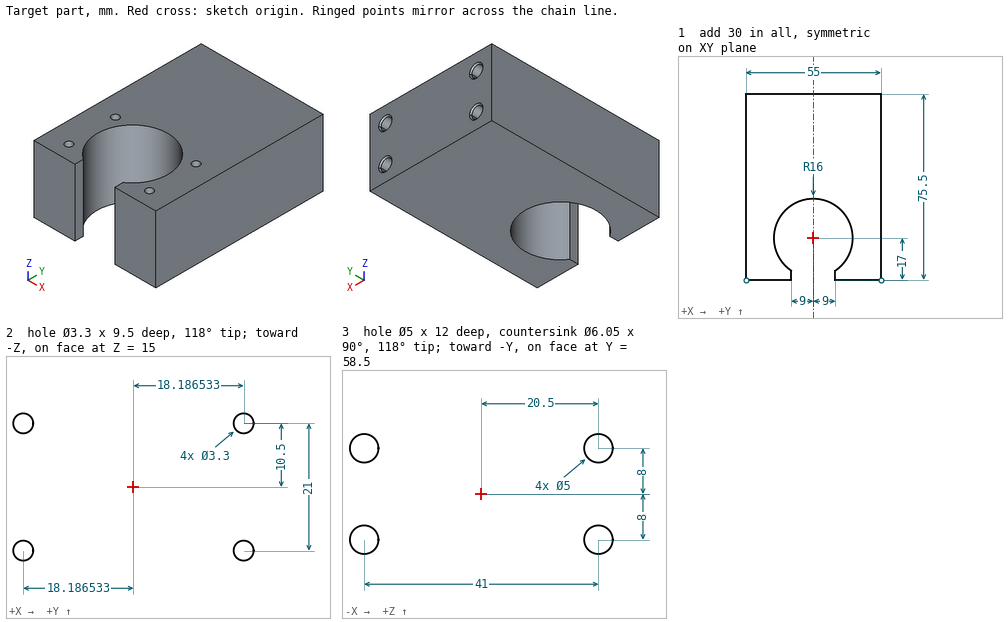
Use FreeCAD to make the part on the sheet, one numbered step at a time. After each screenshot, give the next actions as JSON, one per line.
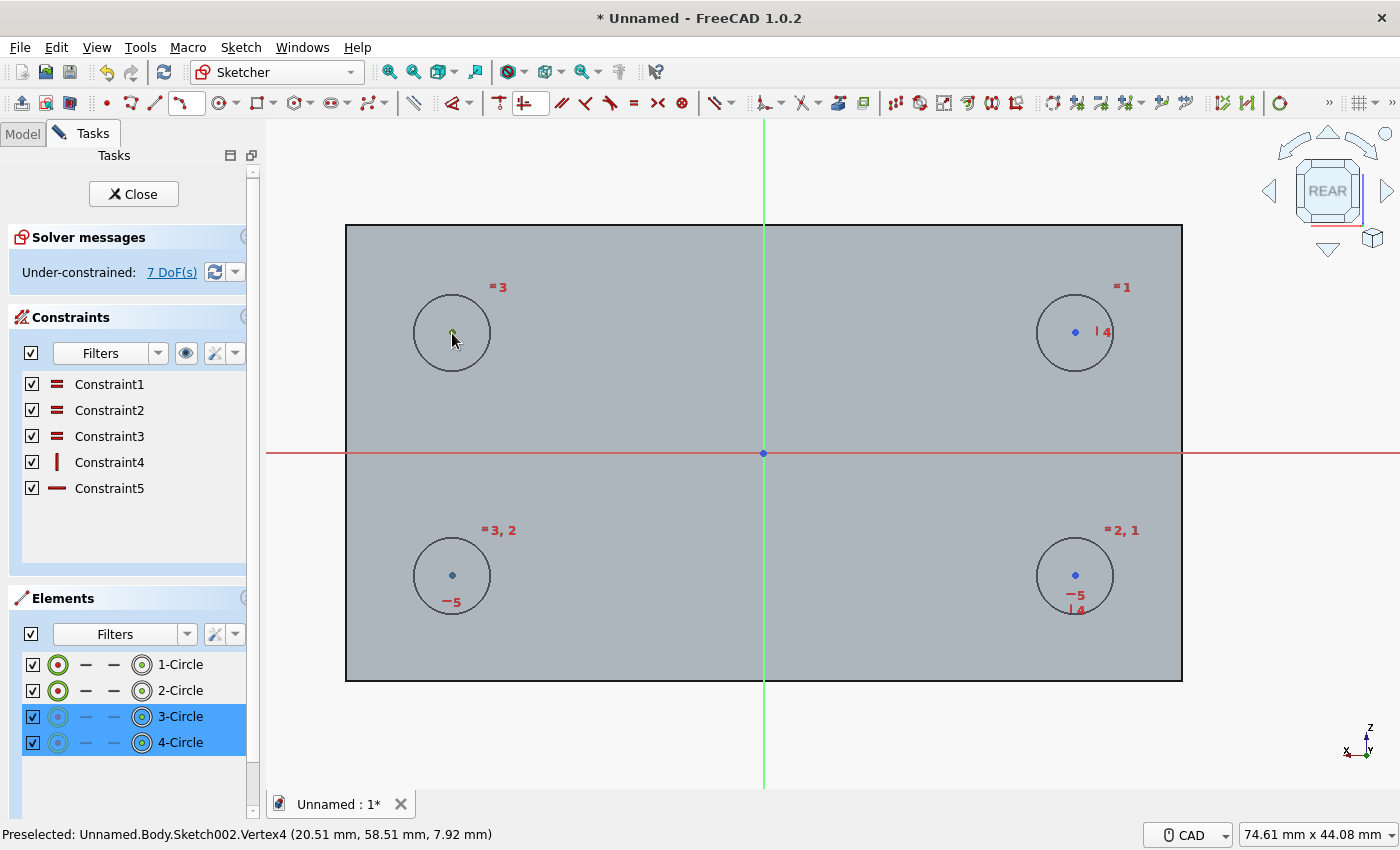
{"action": "left_click", "coordinate": [544, 104]}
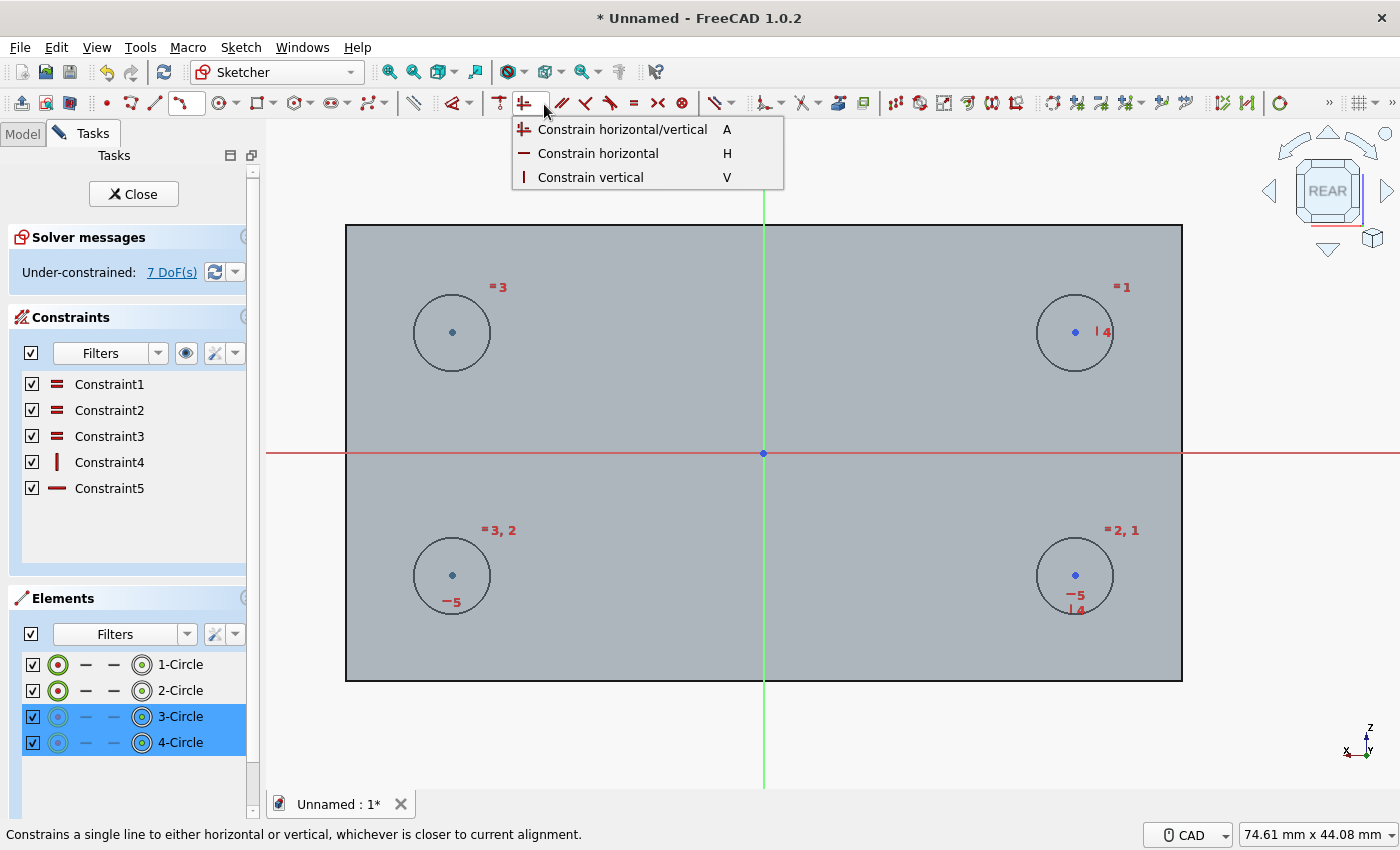
{"action": "left_click", "coordinate": [648, 177]}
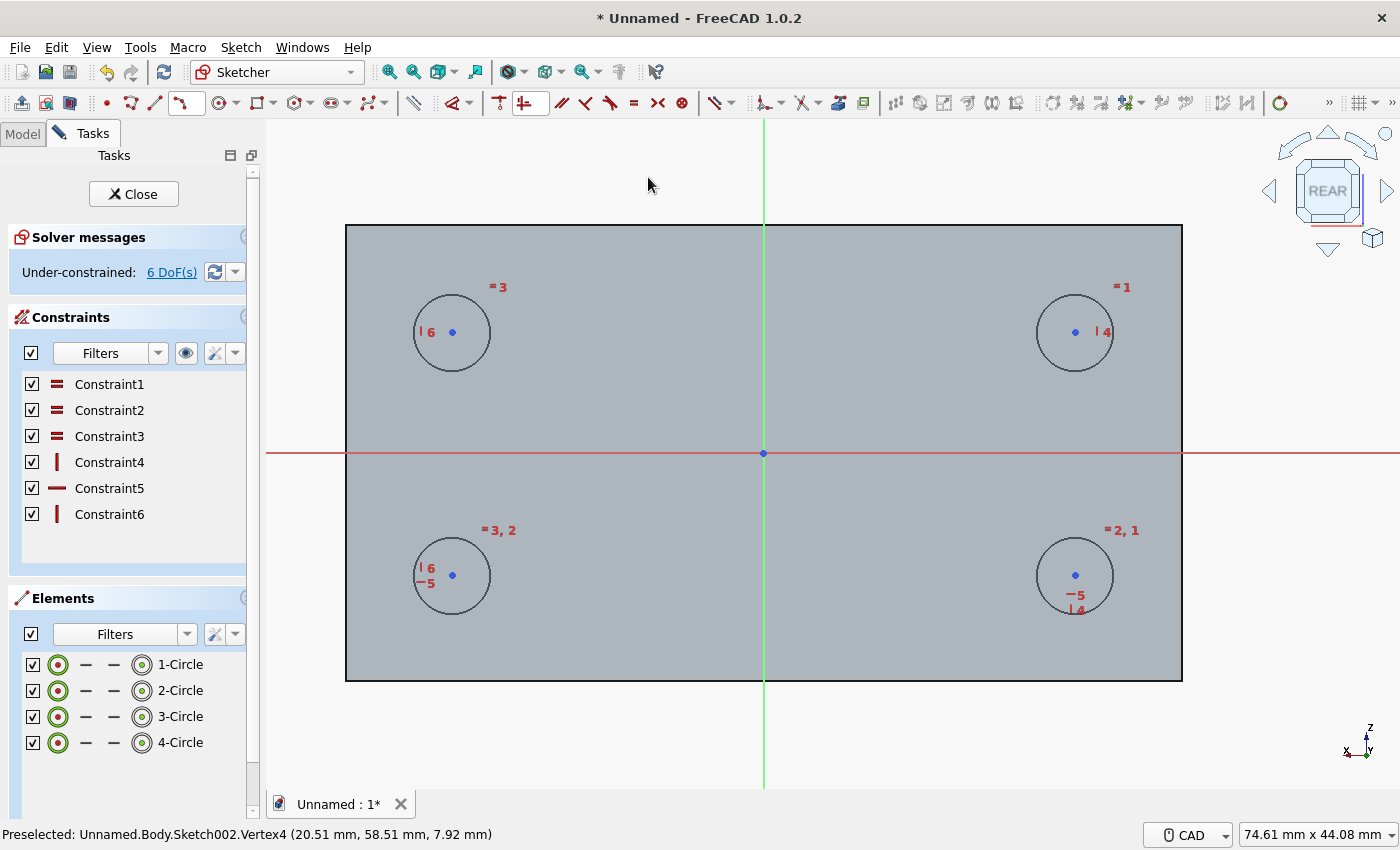
{"action": "left_click", "coordinate": [1075, 333]}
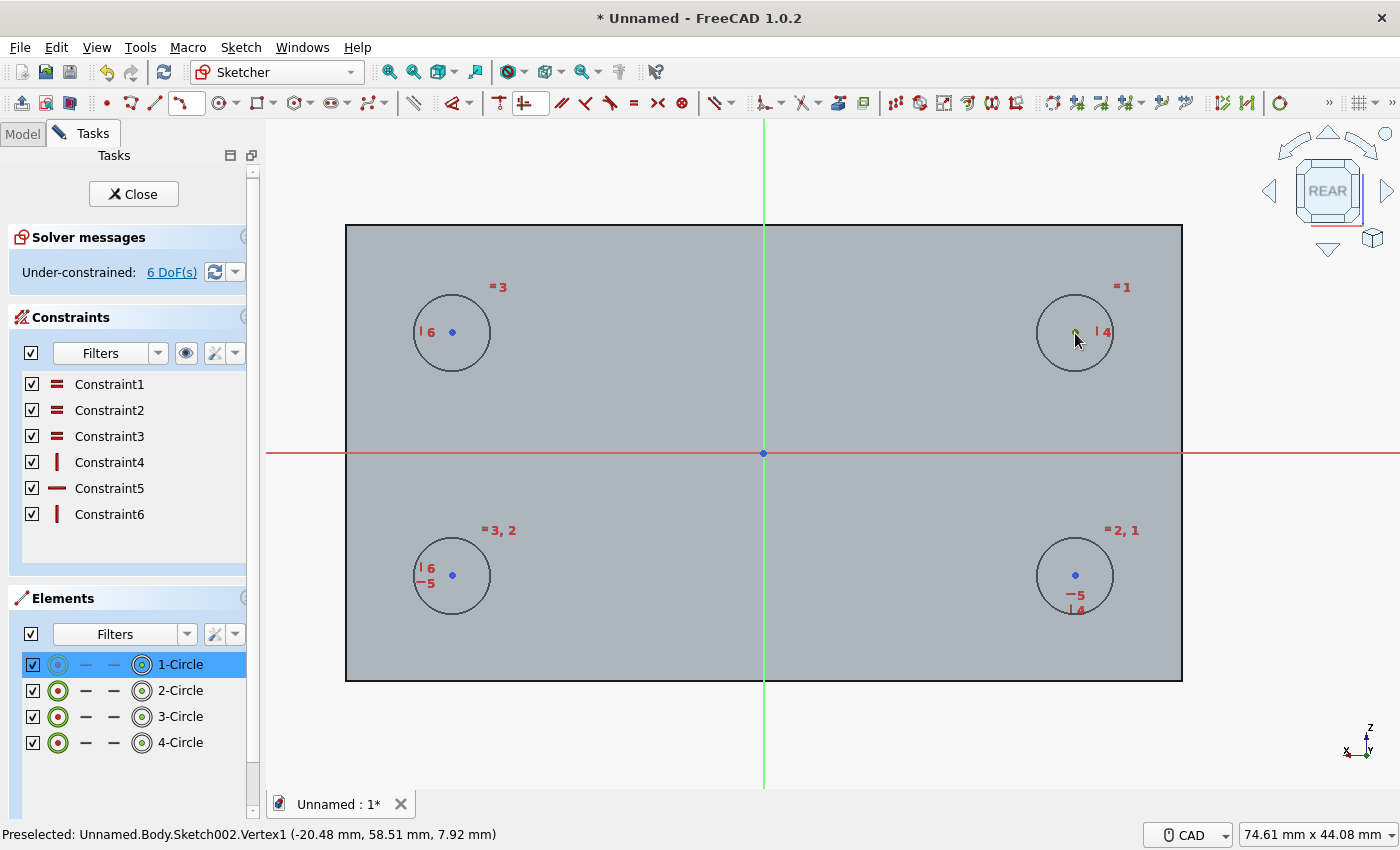
{"action": "left_click", "coordinate": [452, 333]}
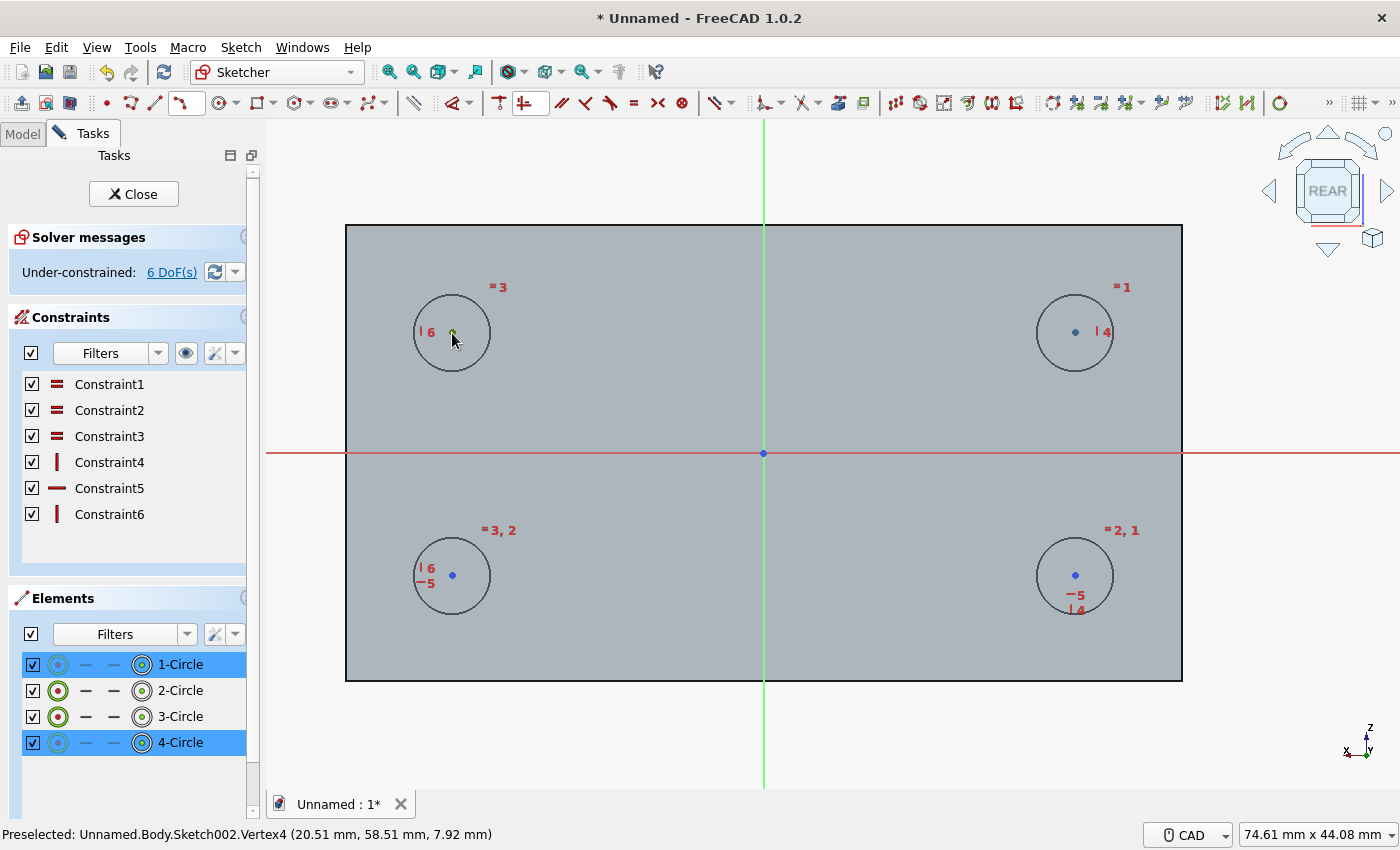
{"action": "key", "text": "h"}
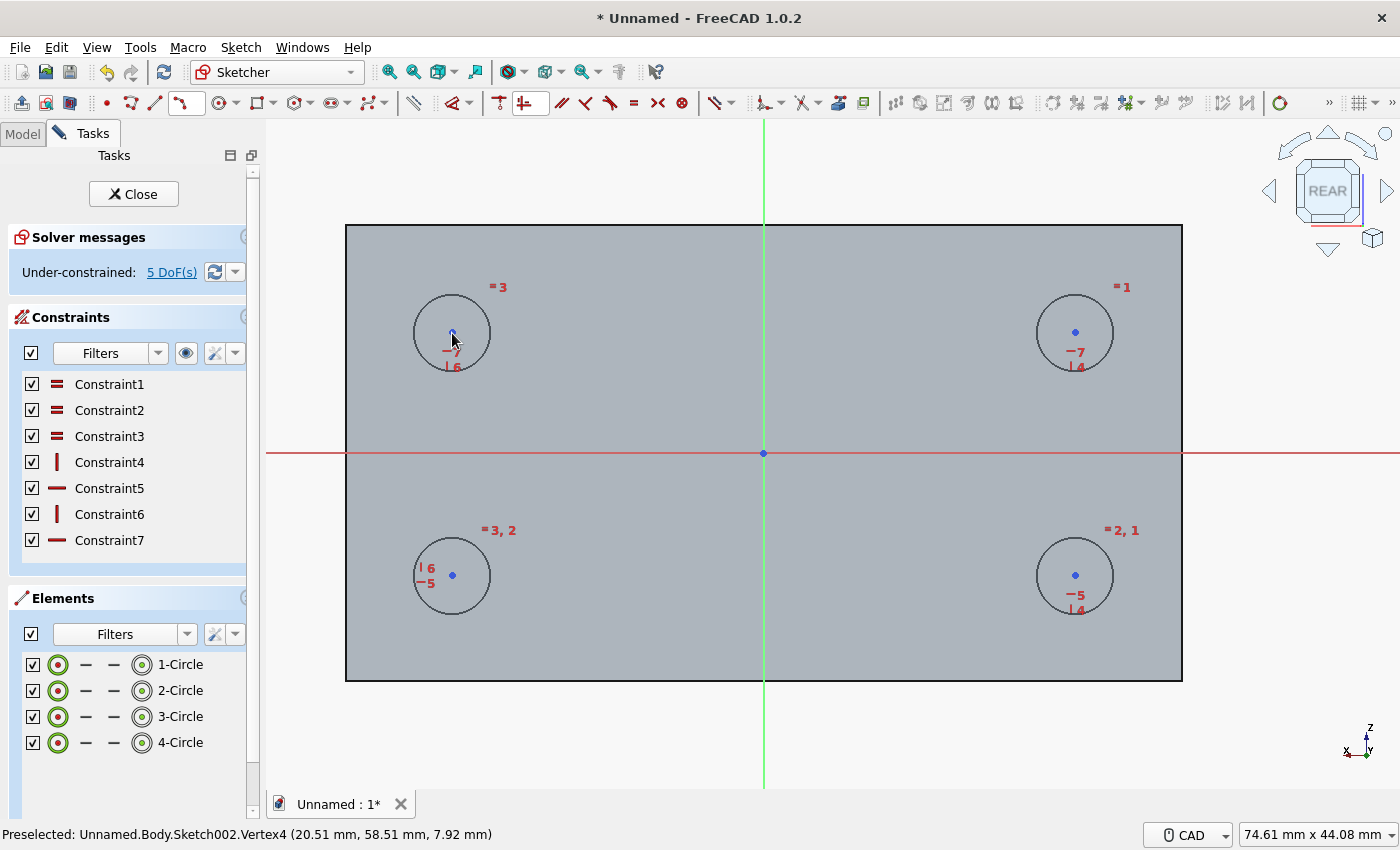
{"action": "left_click", "coordinate": [452, 104]}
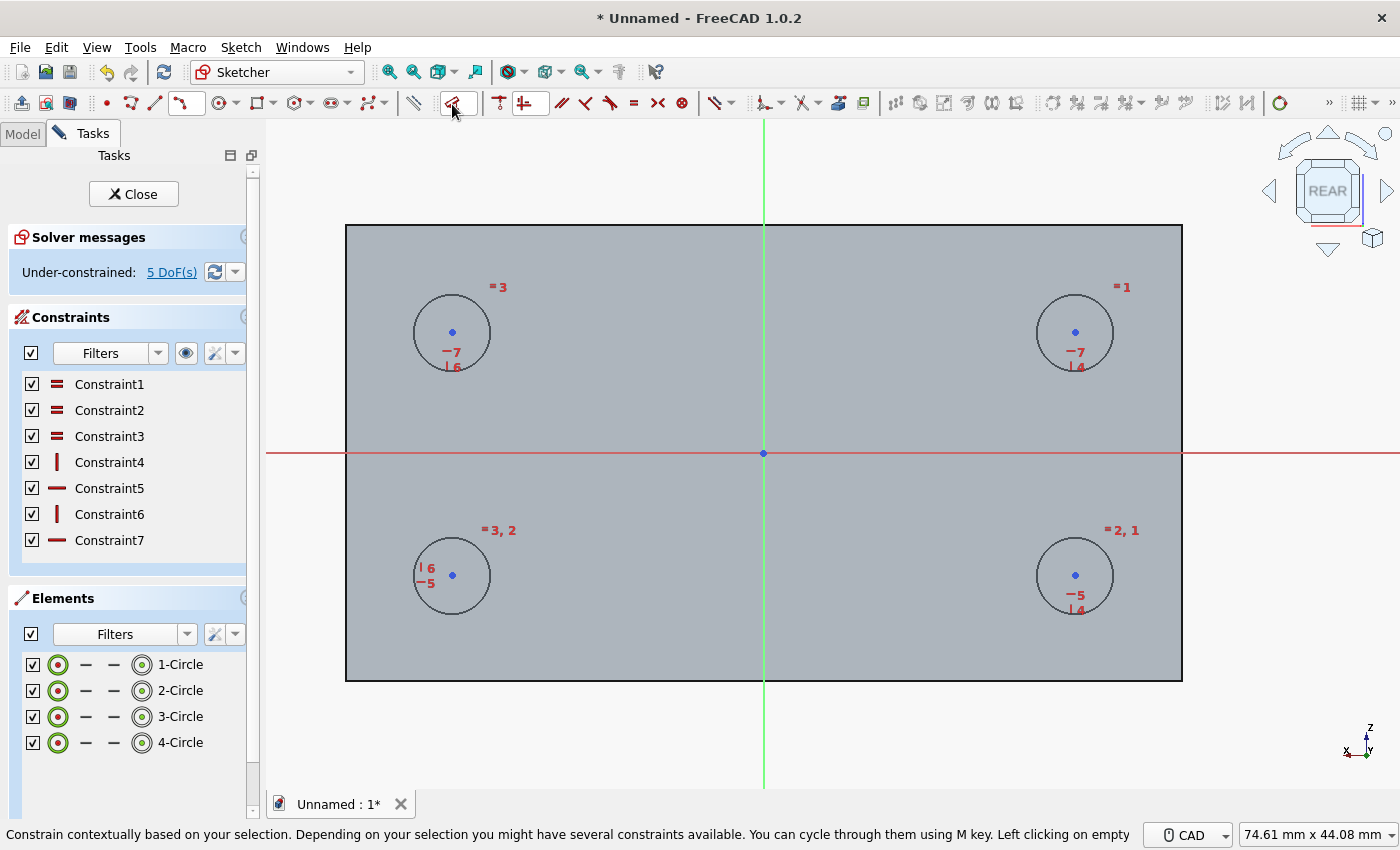
{"action": "left_click", "coordinate": [1102, 306]}
{"action": "left_click", "coordinate": [1125, 283]}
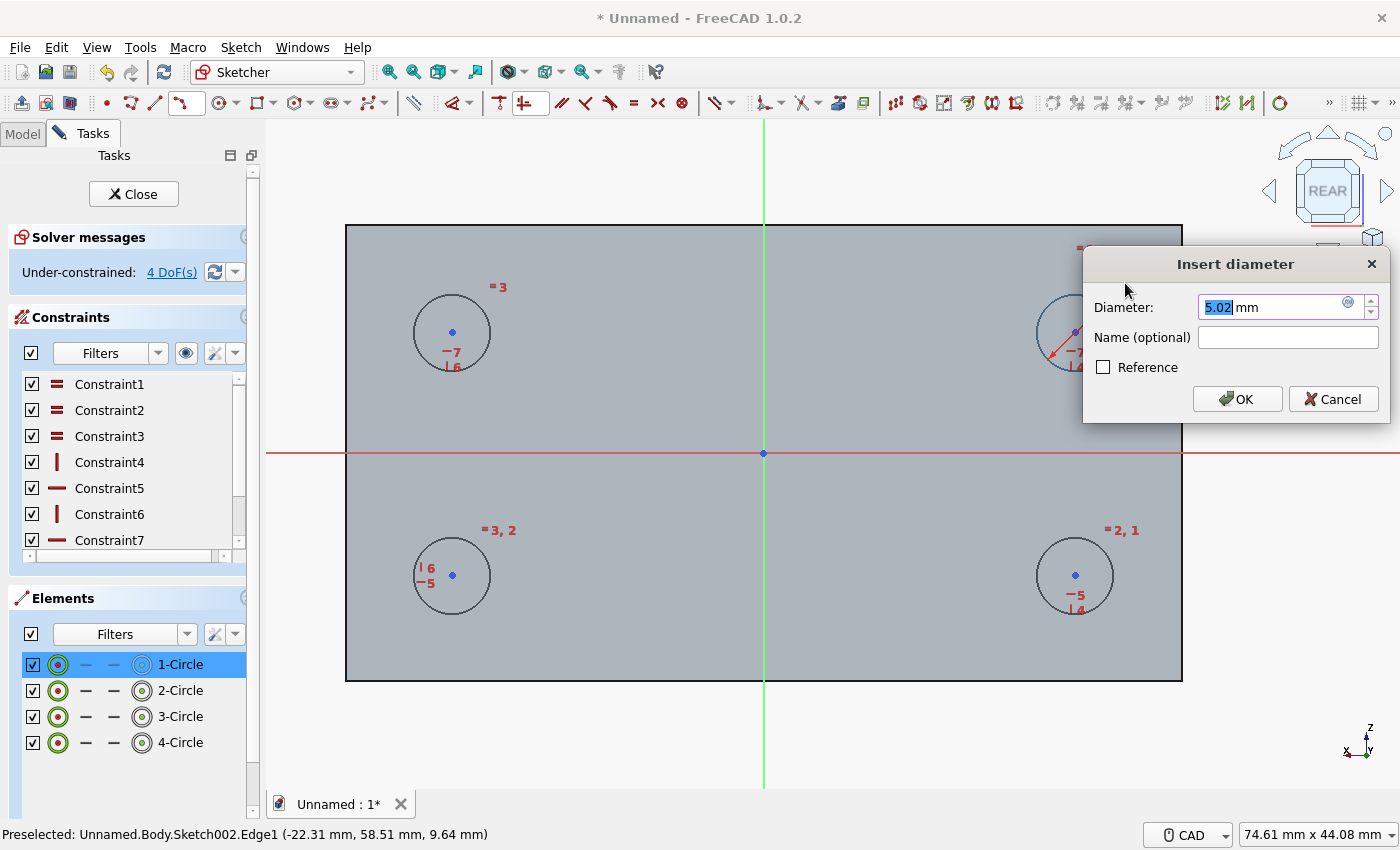
{"action": "type", "text": "5"}
{"action": "key", "text": "Return"}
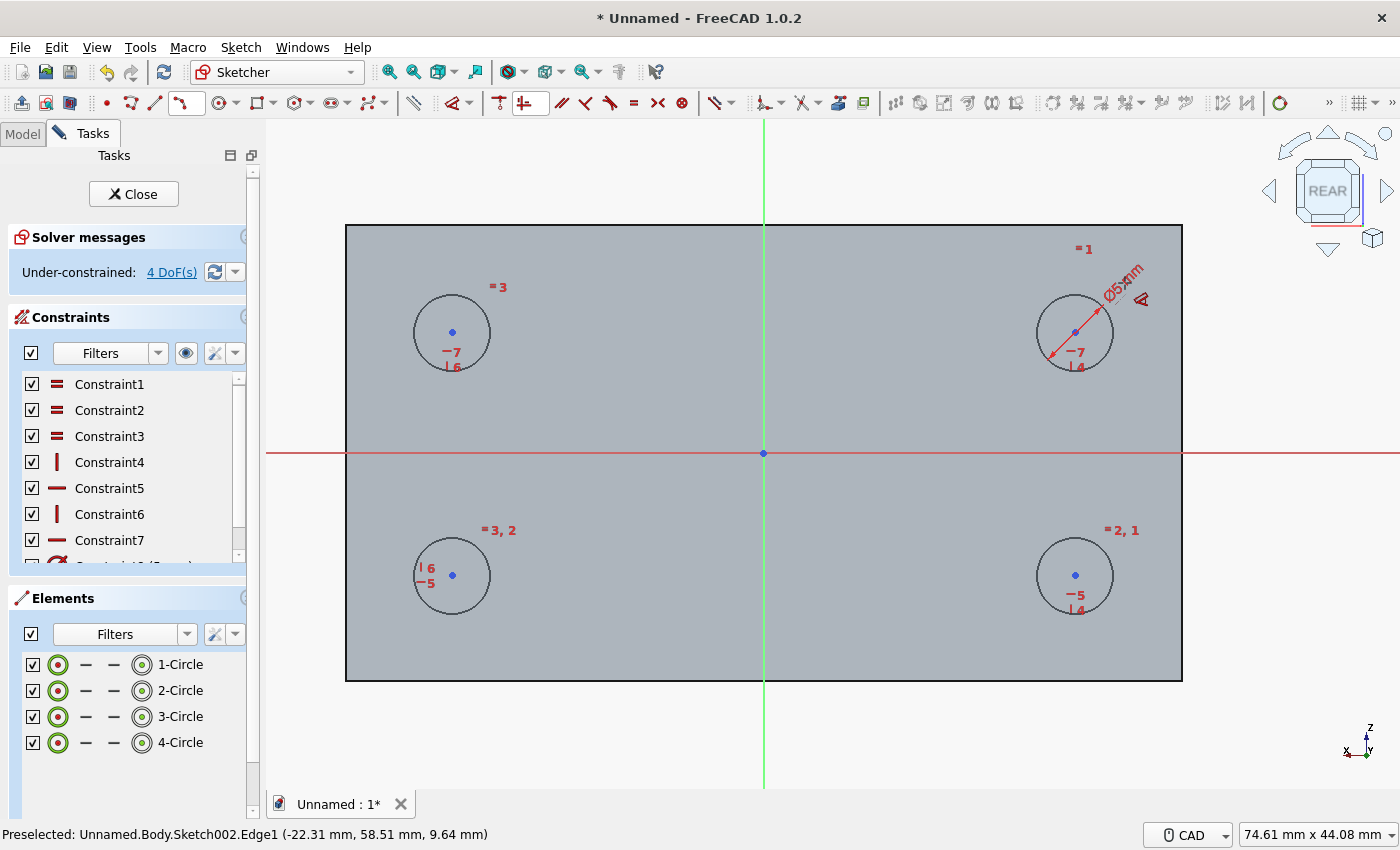
{"action": "left_click", "coordinate": [1075, 333]}
{"action": "left_click", "coordinate": [1109, 393]}